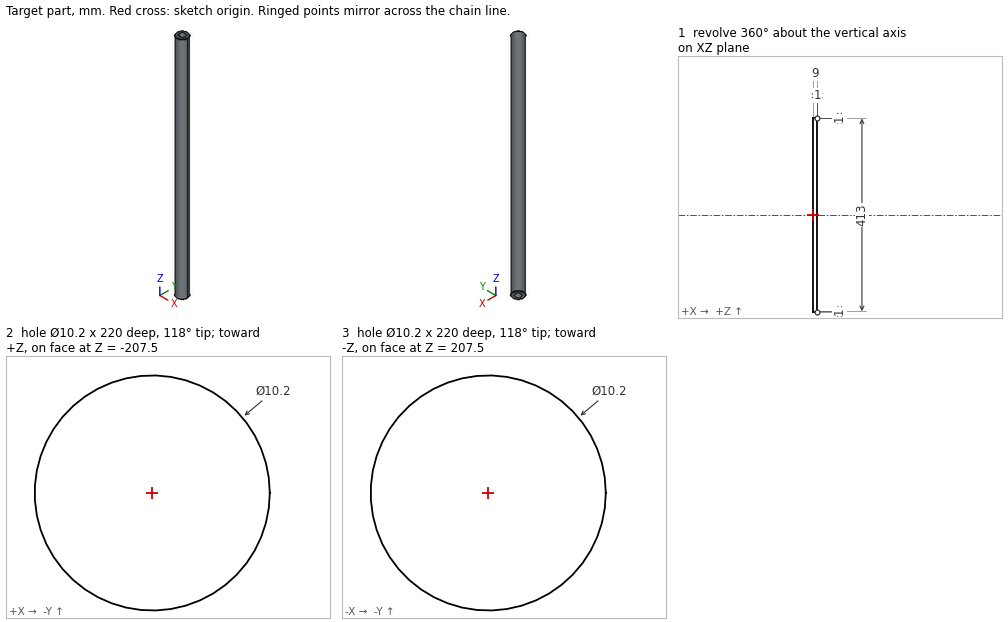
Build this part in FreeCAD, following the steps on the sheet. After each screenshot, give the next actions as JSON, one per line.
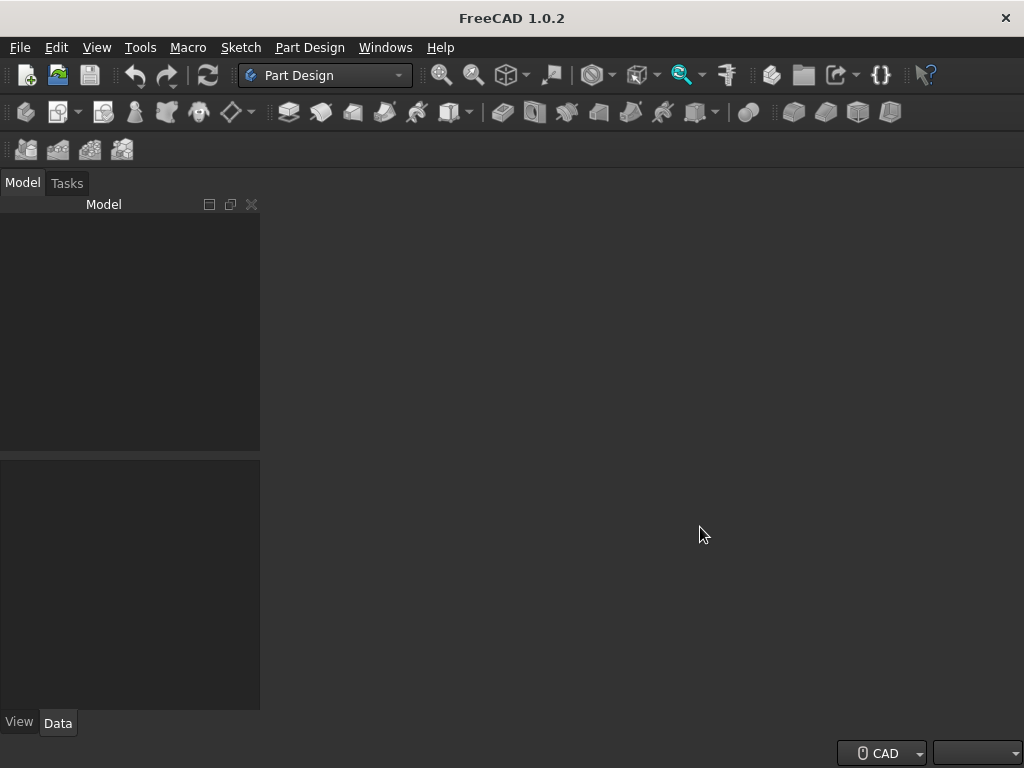
{"action": "key", "text": "ctrl+n"}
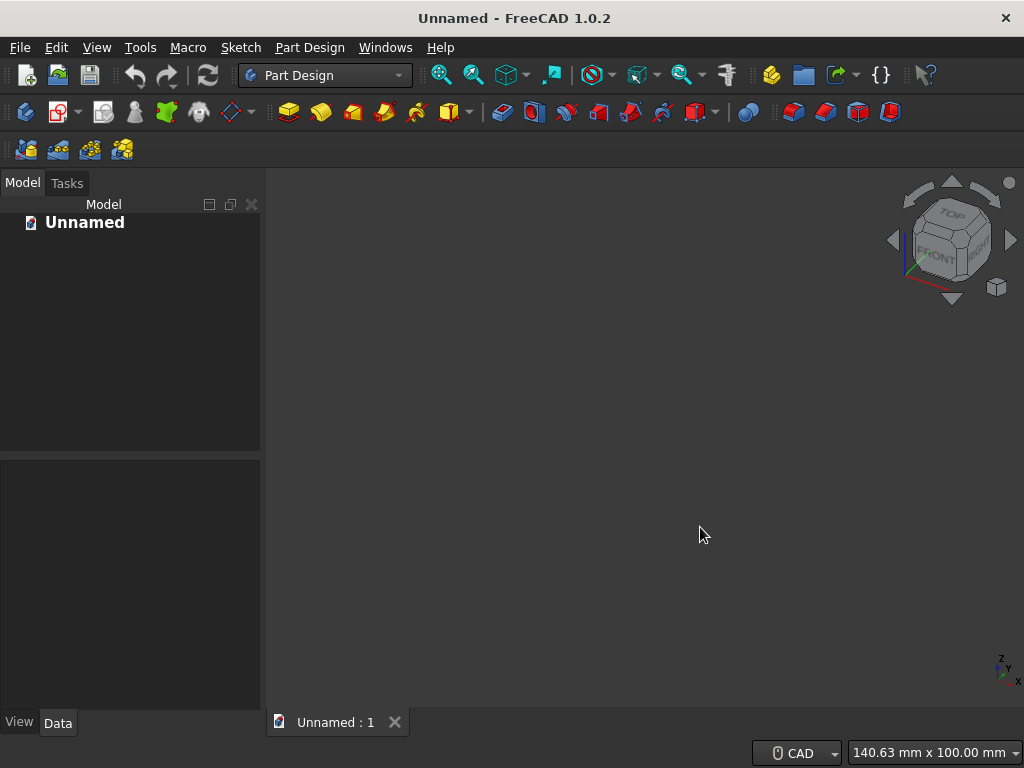
{"action": "left_click", "coordinate": [58, 112]}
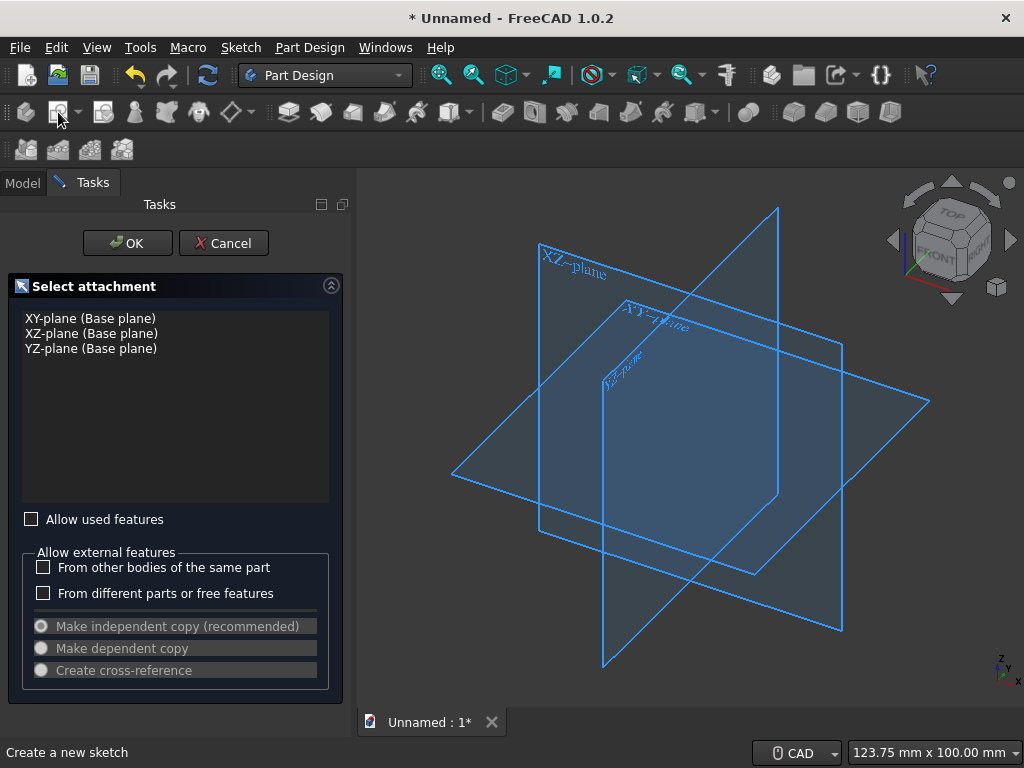
{"action": "left_click", "coordinate": [82, 334]}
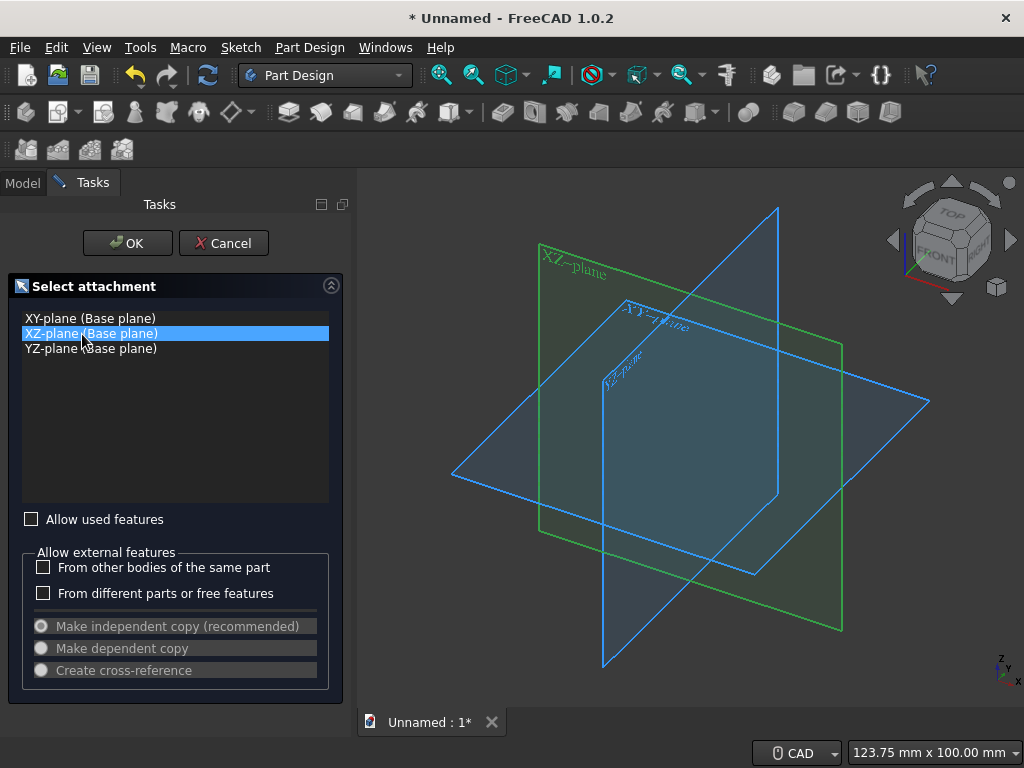
{"action": "left_click", "coordinate": [128, 243]}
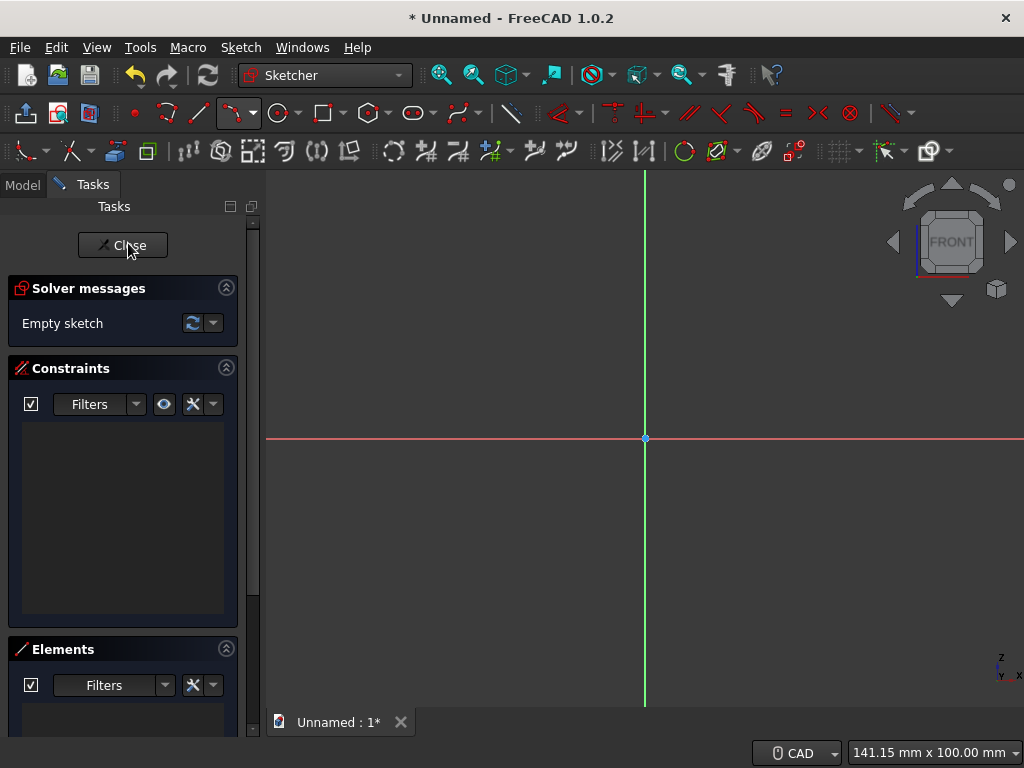
{"action": "scroll", "coordinate": [558, 438], "scroll_direction": "down", "scroll_amount": 9}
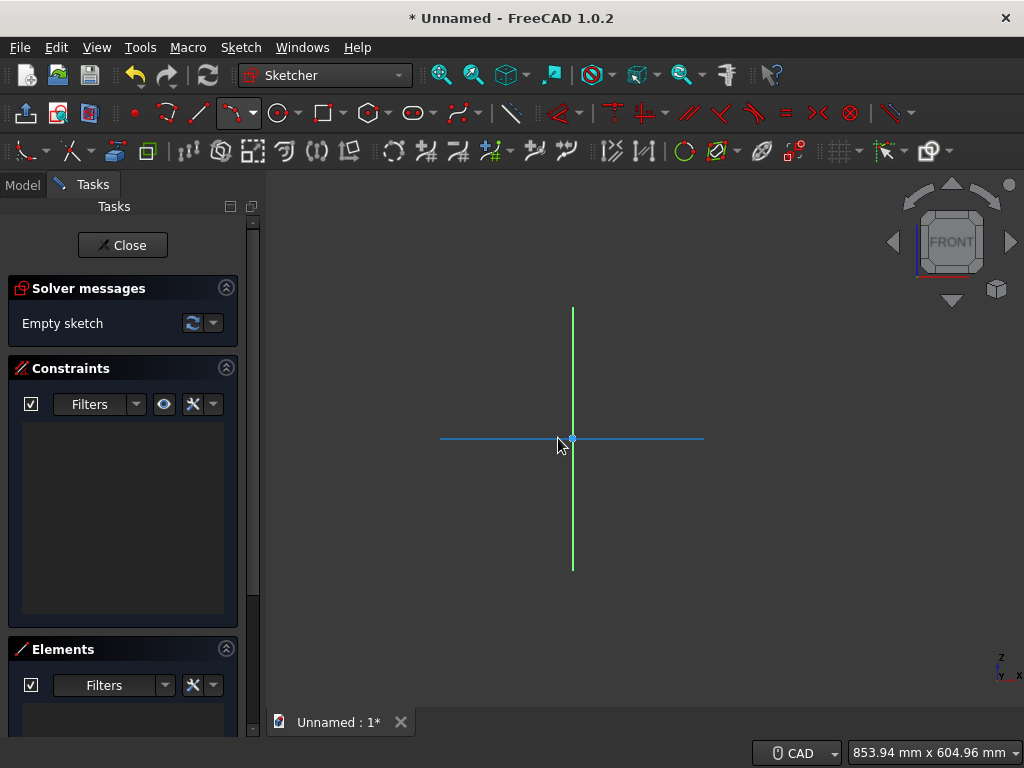
{"action": "left_click", "coordinate": [168, 114]}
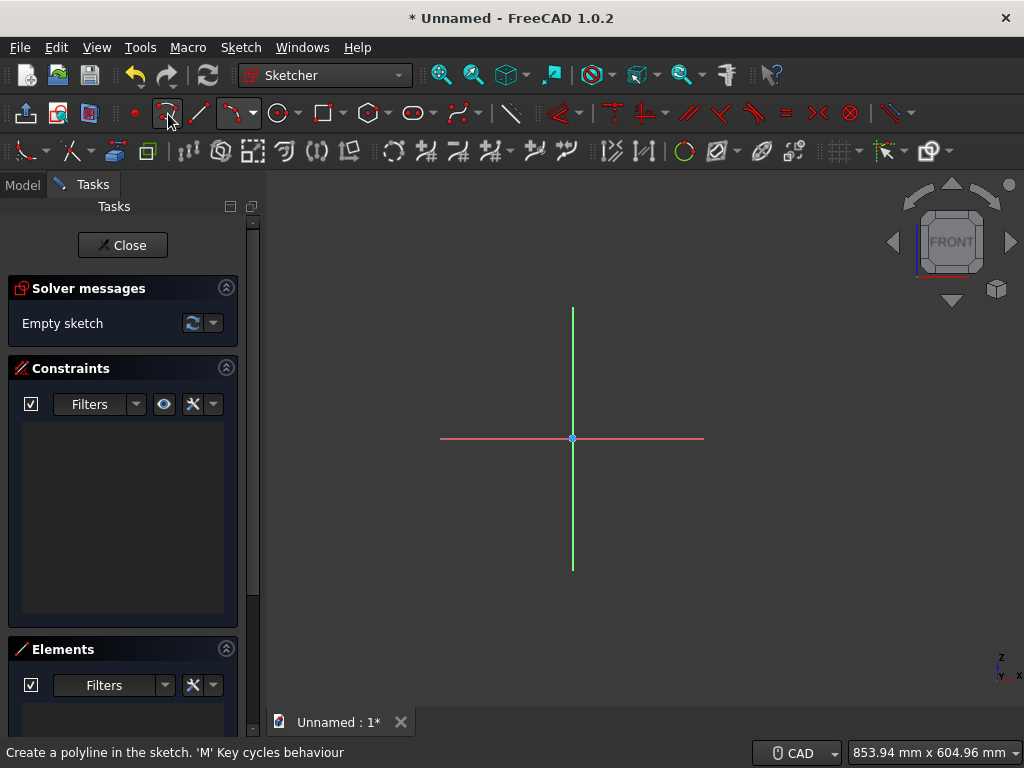
{"action": "scroll", "coordinate": [582, 622], "scroll_direction": "up", "scroll_amount": 3}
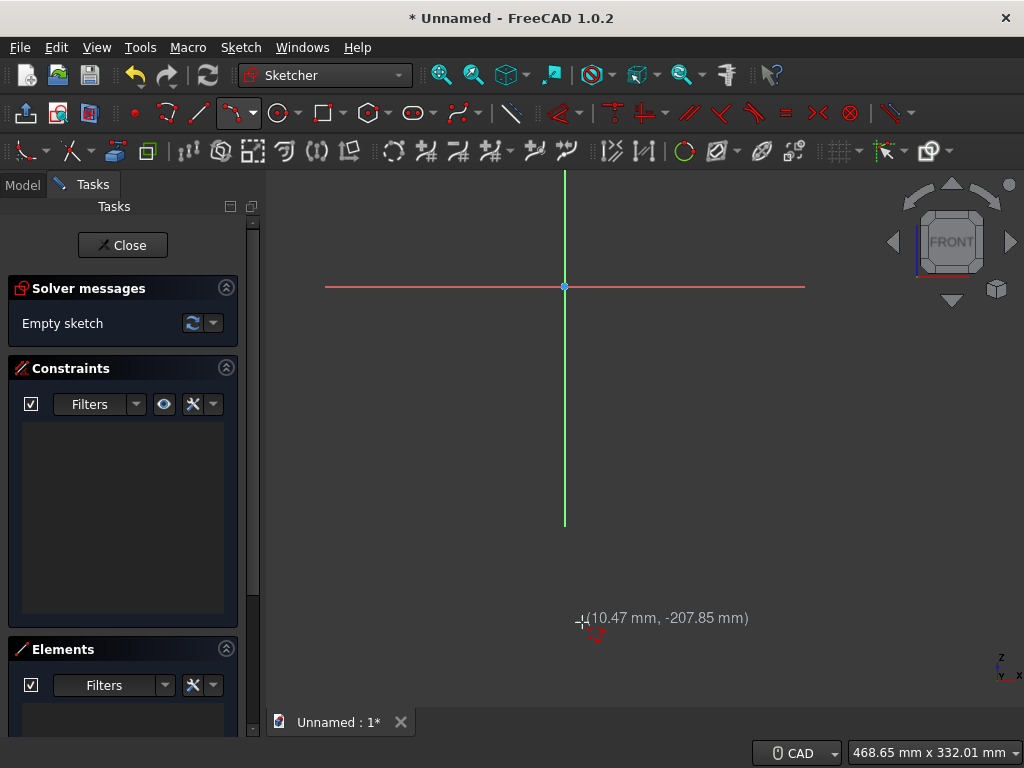
{"action": "left_click", "coordinate": [581, 621]}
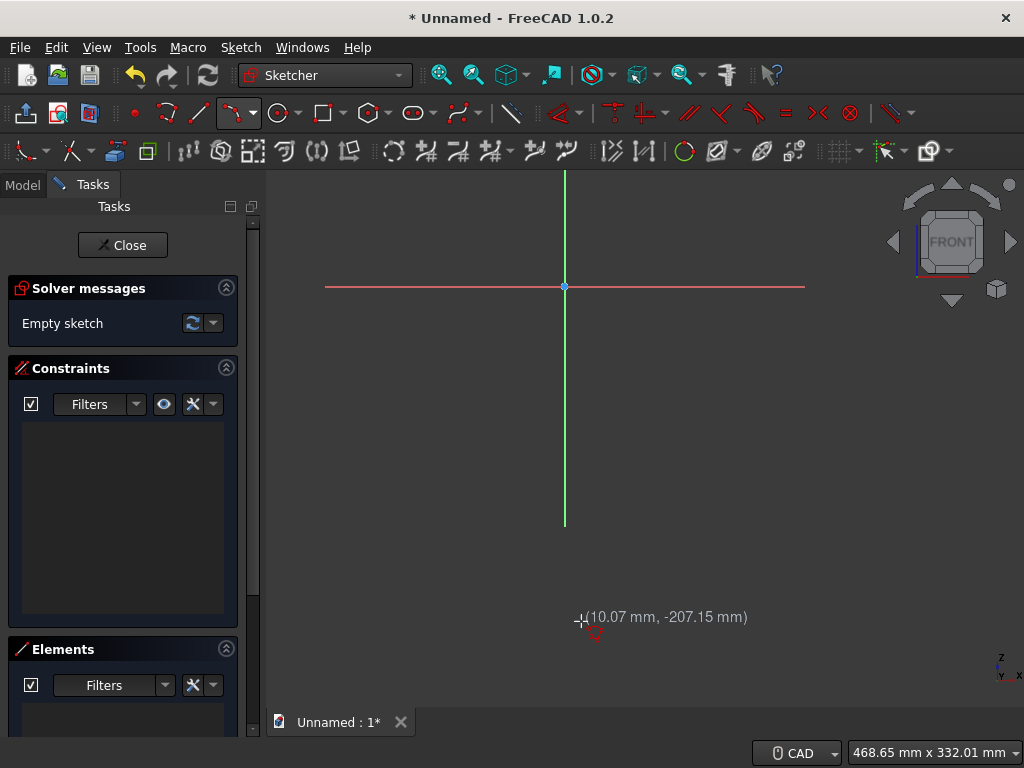
{"action": "scroll", "coordinate": [581, 623], "scroll_direction": "down", "scroll_amount": 3}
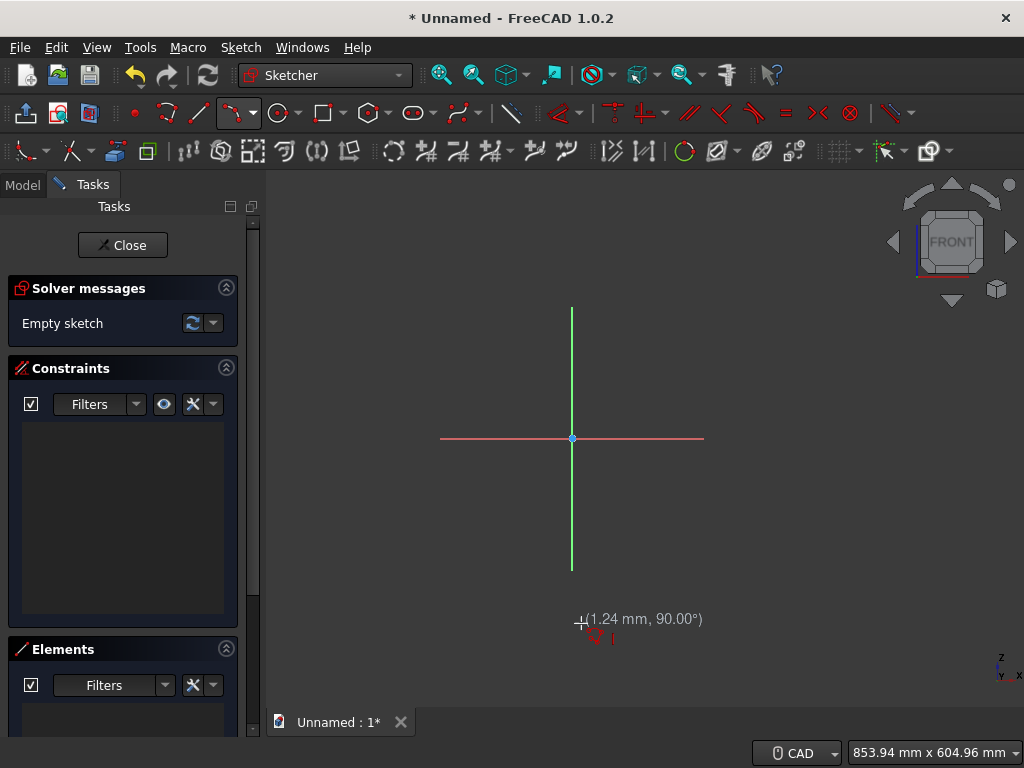
{"action": "scroll", "coordinate": [581, 256], "scroll_direction": "up", "scroll_amount": 3}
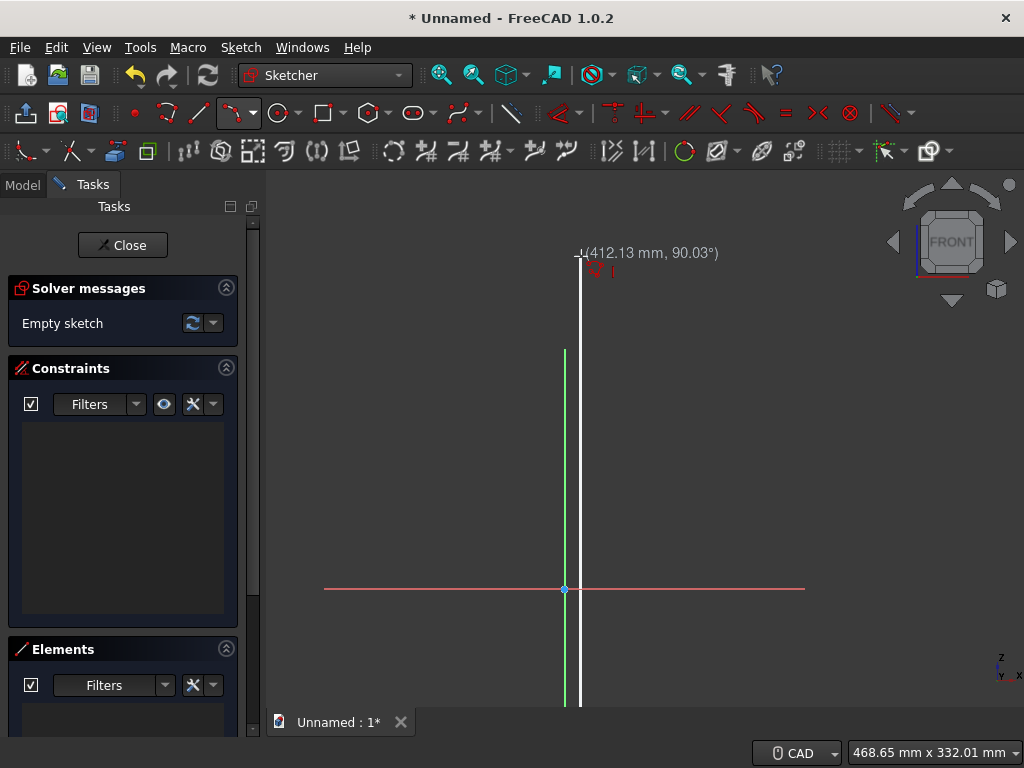
{"action": "left_click", "coordinate": [581, 255]}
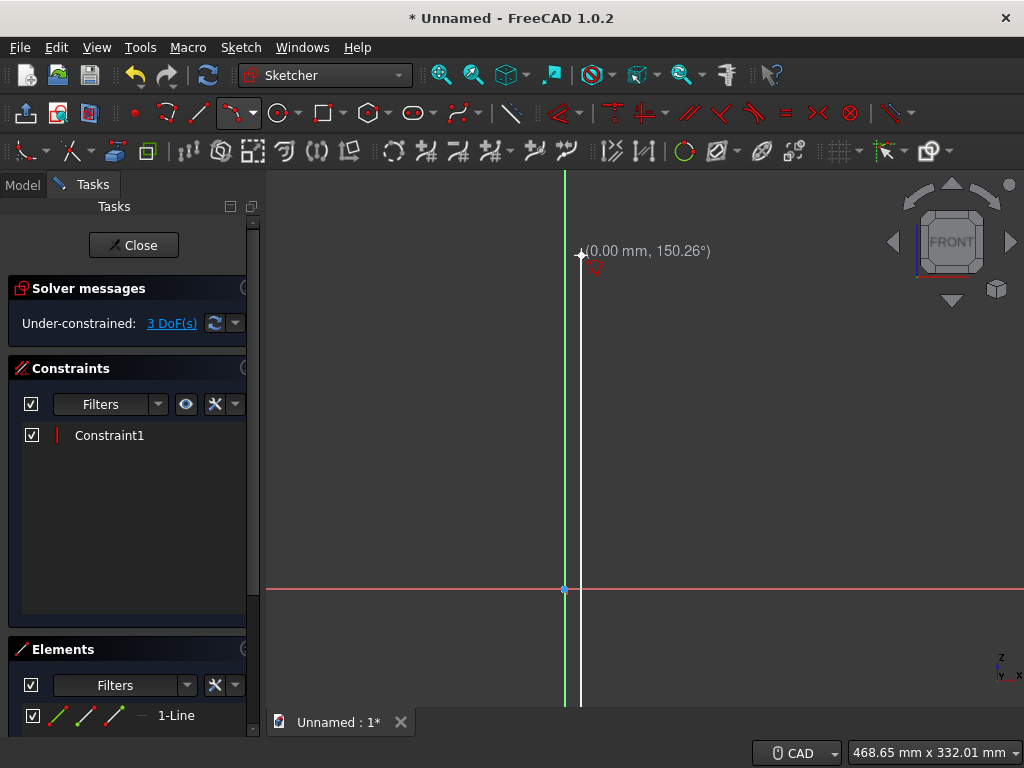
{"action": "scroll", "coordinate": [579, 254], "scroll_direction": "up", "scroll_amount": 10}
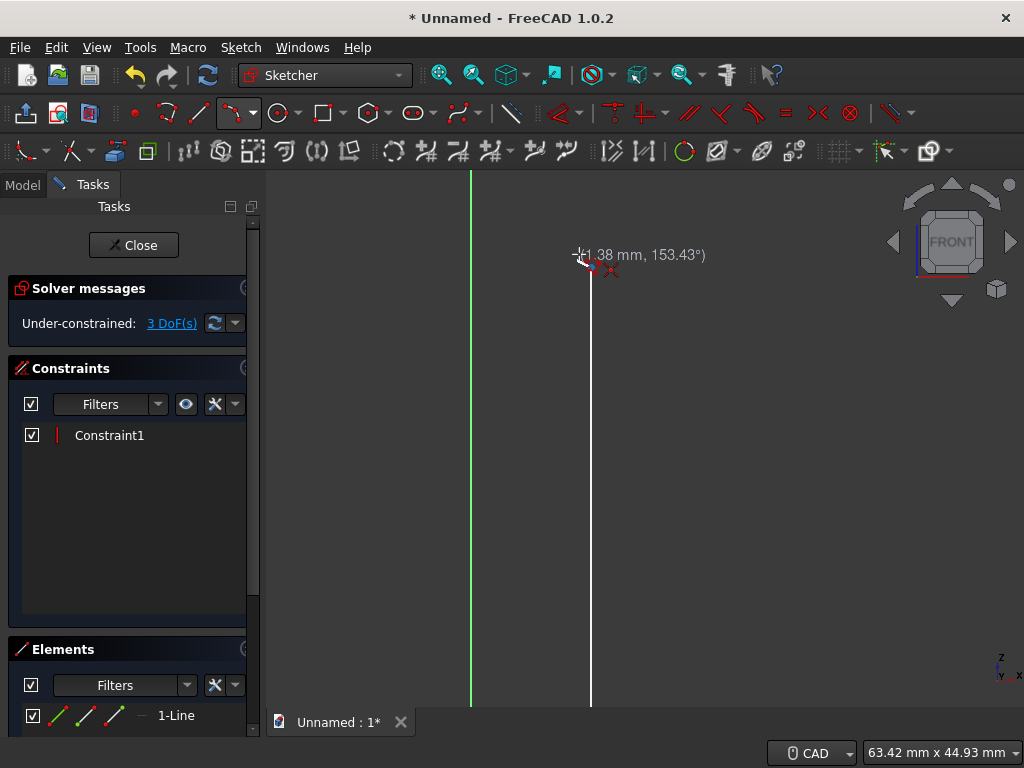
{"action": "left_click", "coordinate": [578, 250]}